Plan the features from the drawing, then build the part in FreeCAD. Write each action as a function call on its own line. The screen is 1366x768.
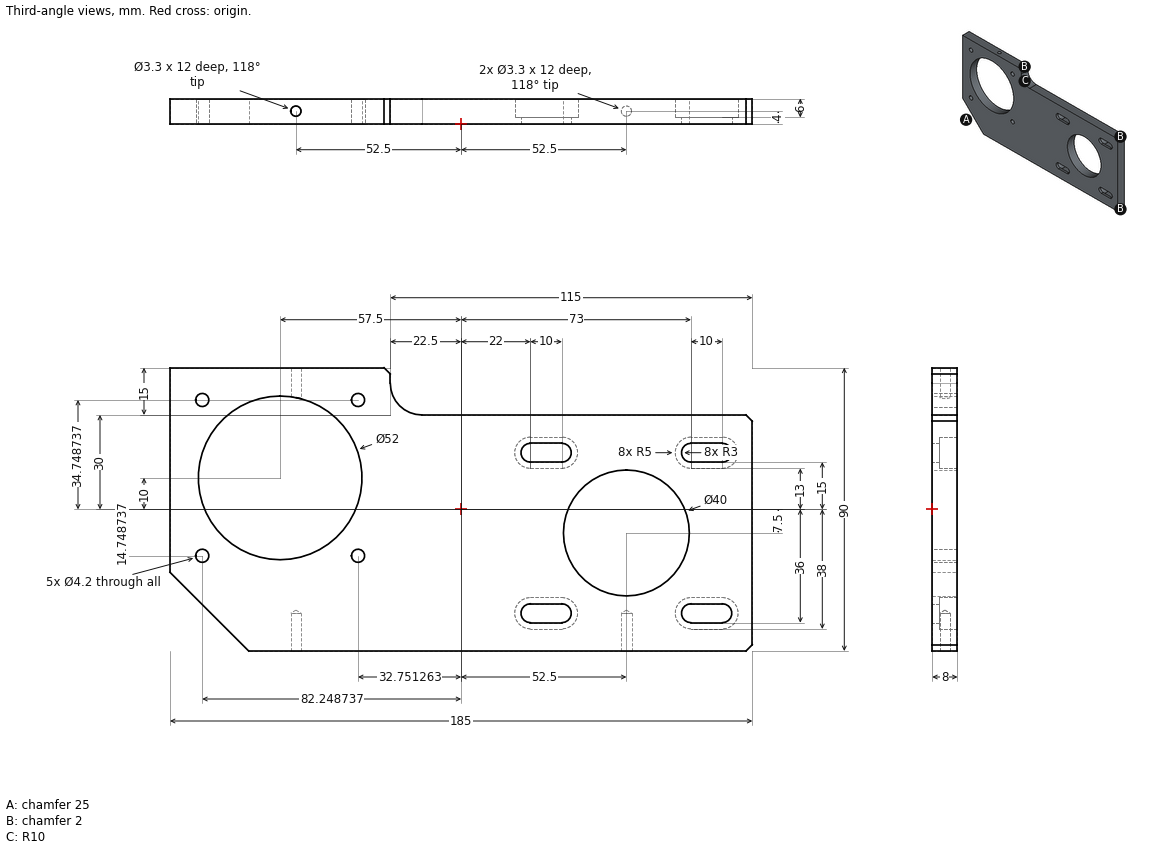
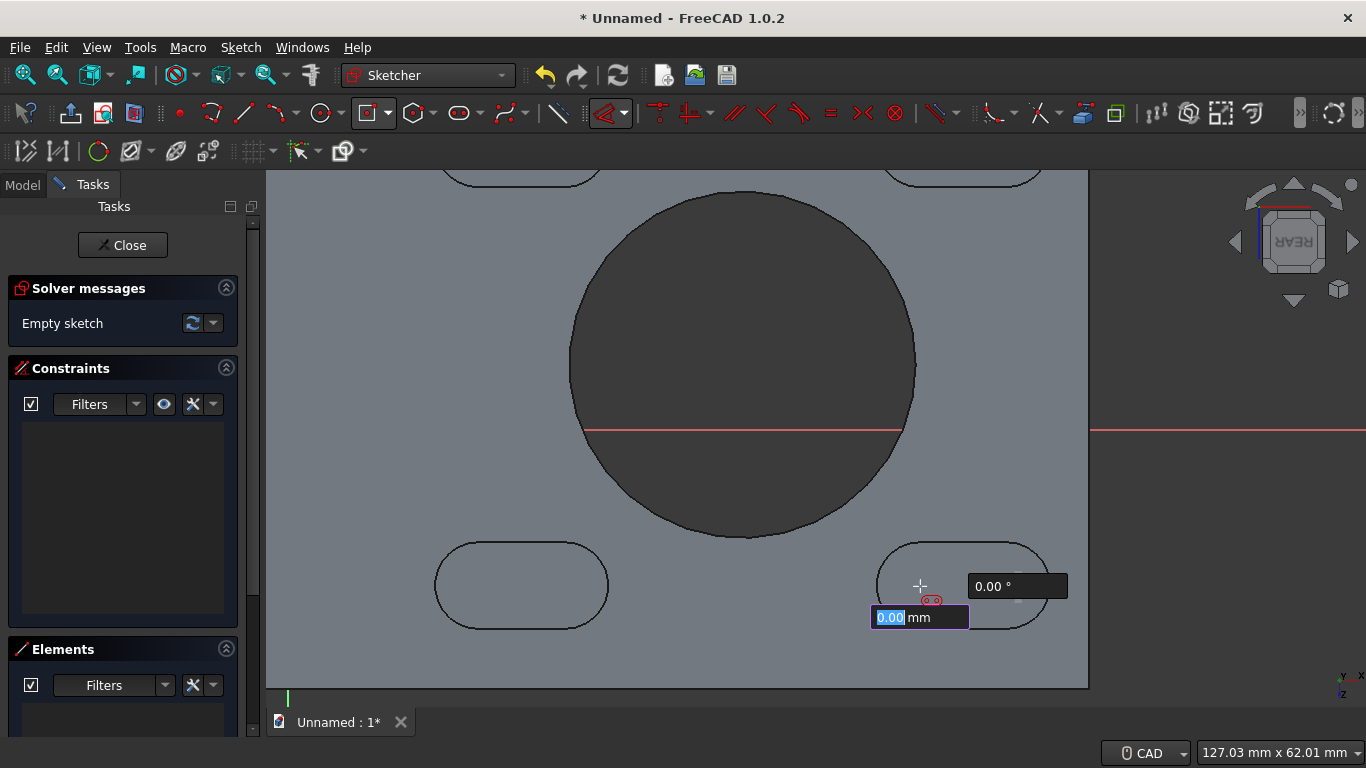
click(1007, 586)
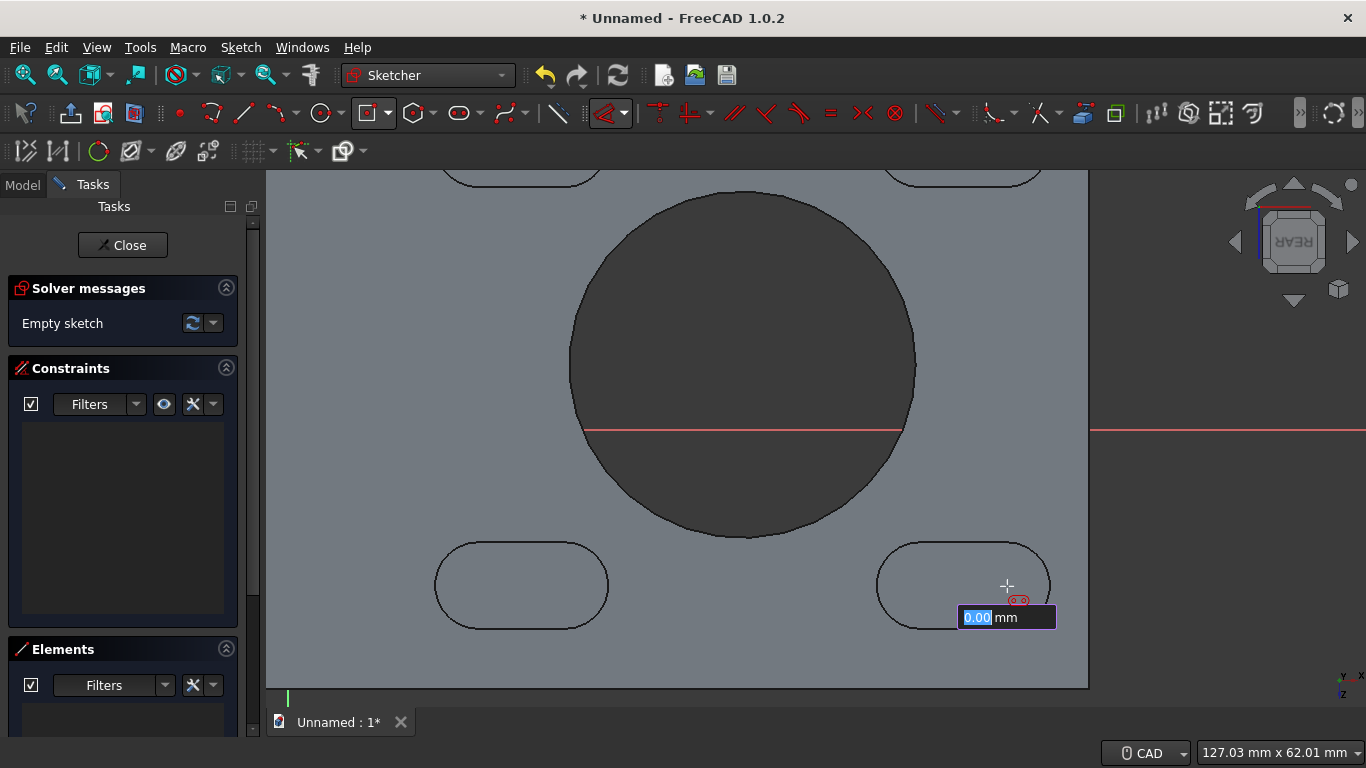
click(963, 560)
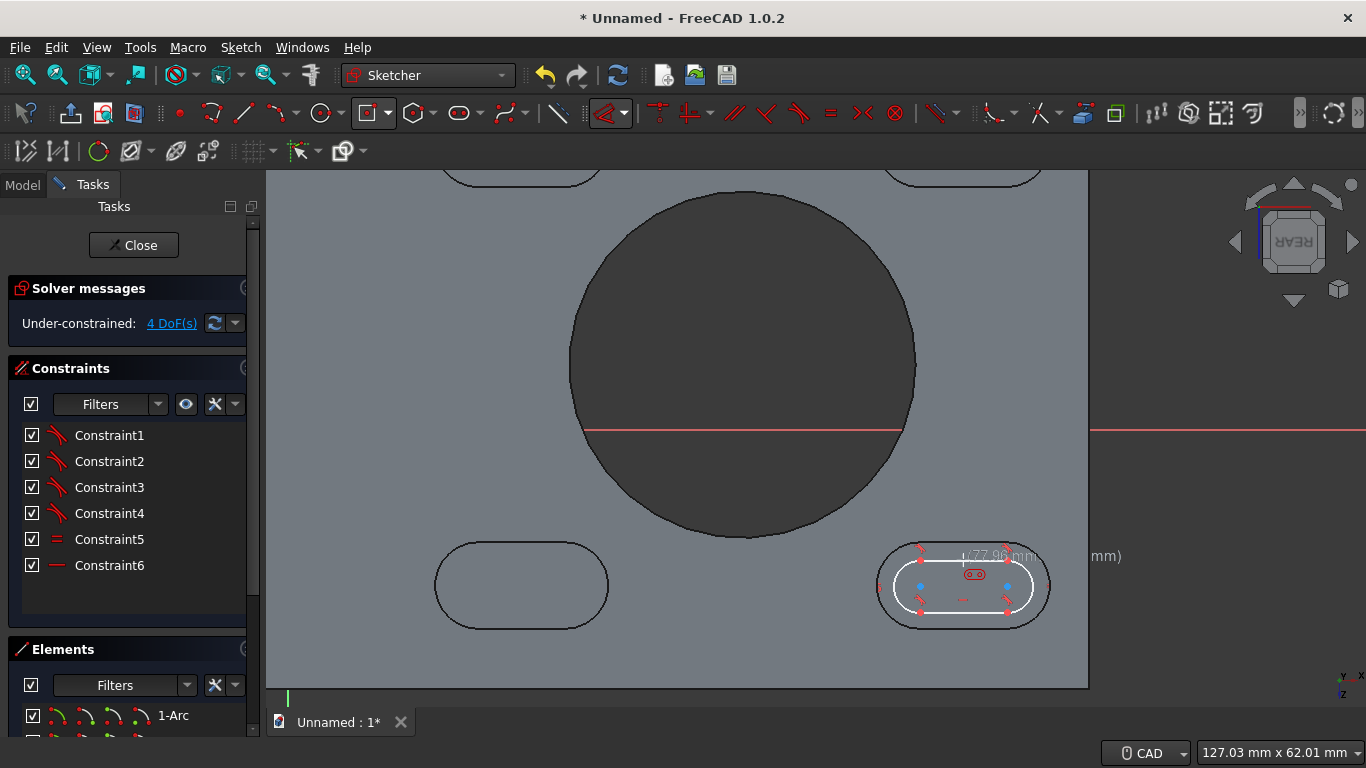
scroll(925, 588, down, 2)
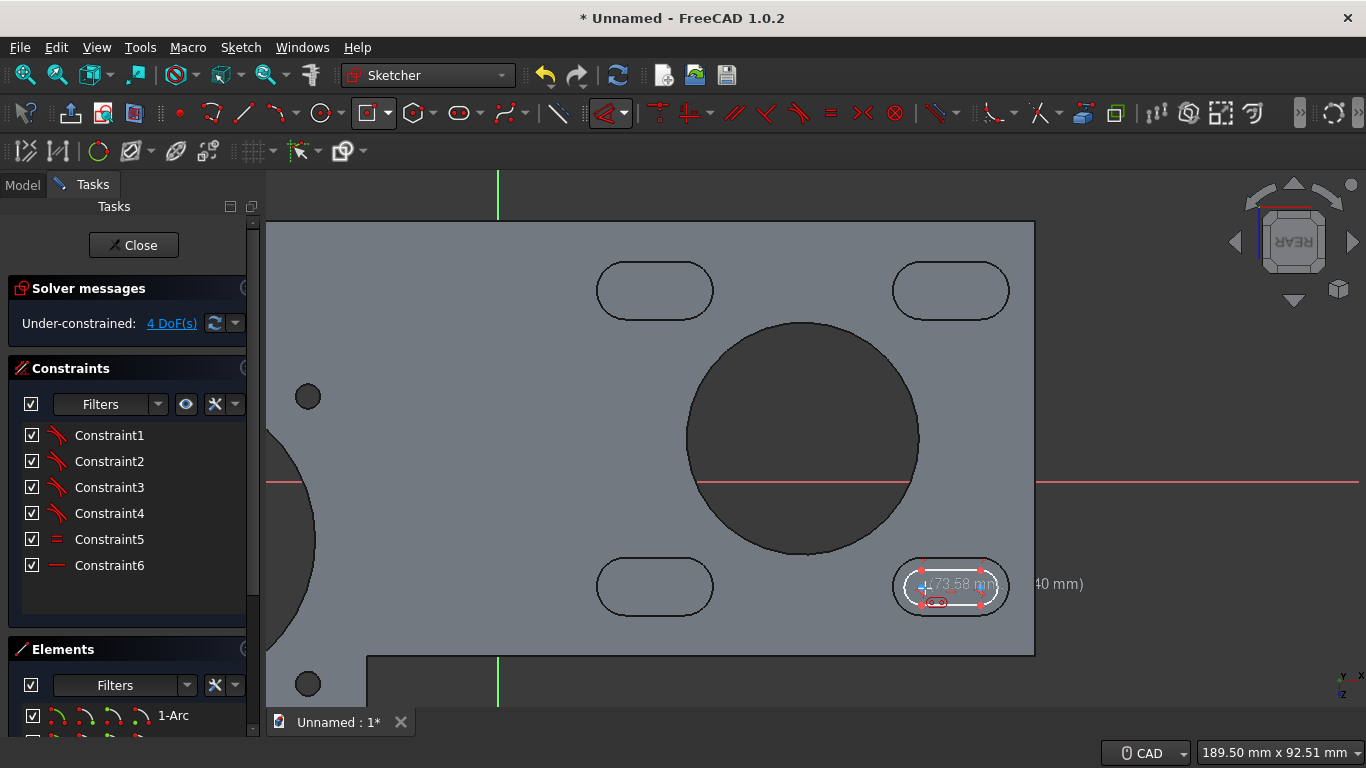
scroll(922, 291, up, 2)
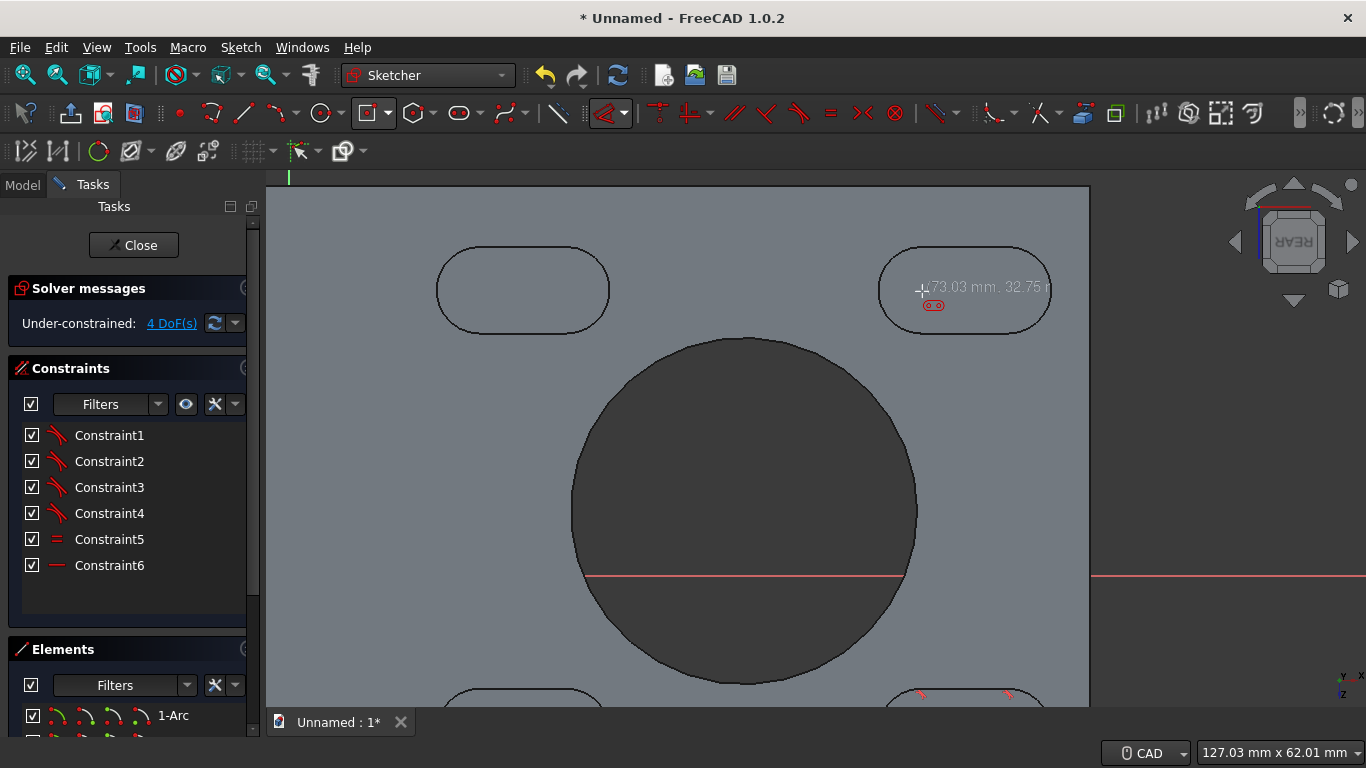
click(921, 290)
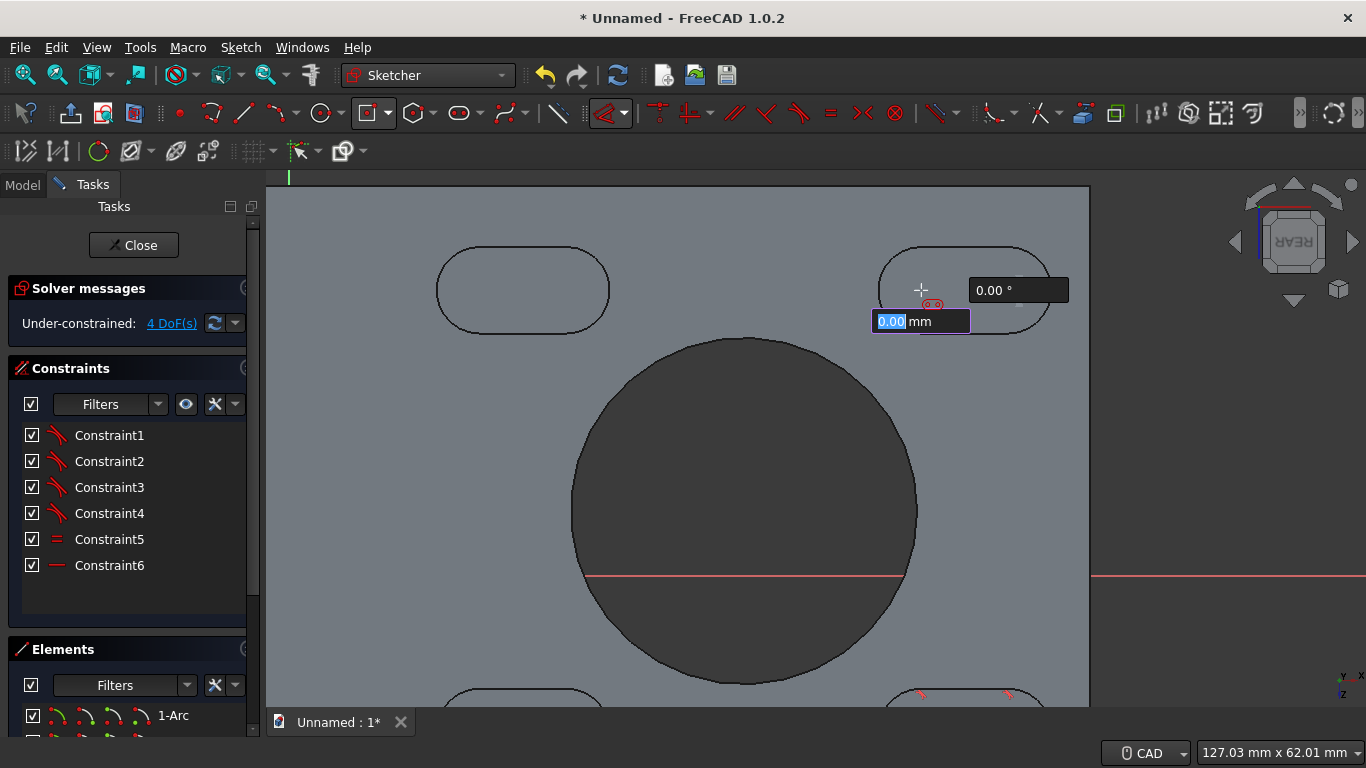
click(1008, 290)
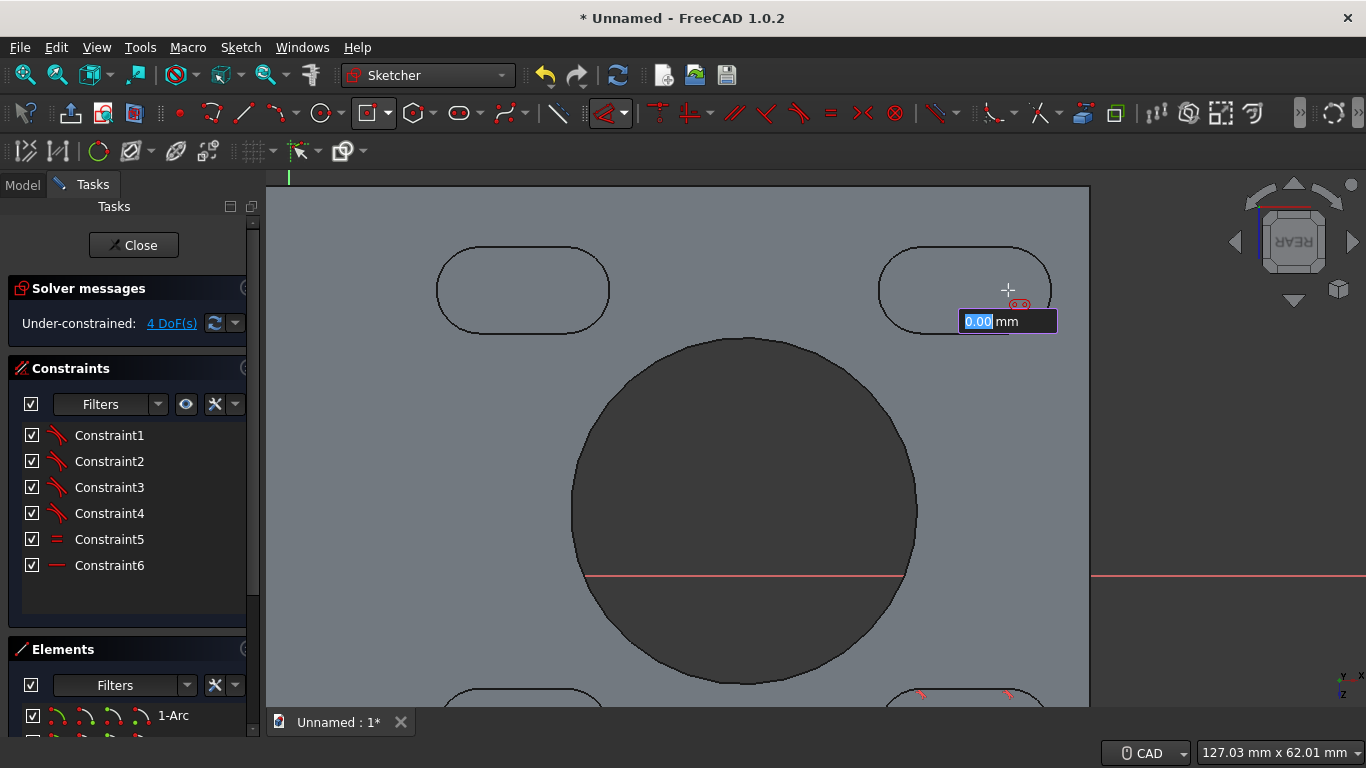
click(965, 316)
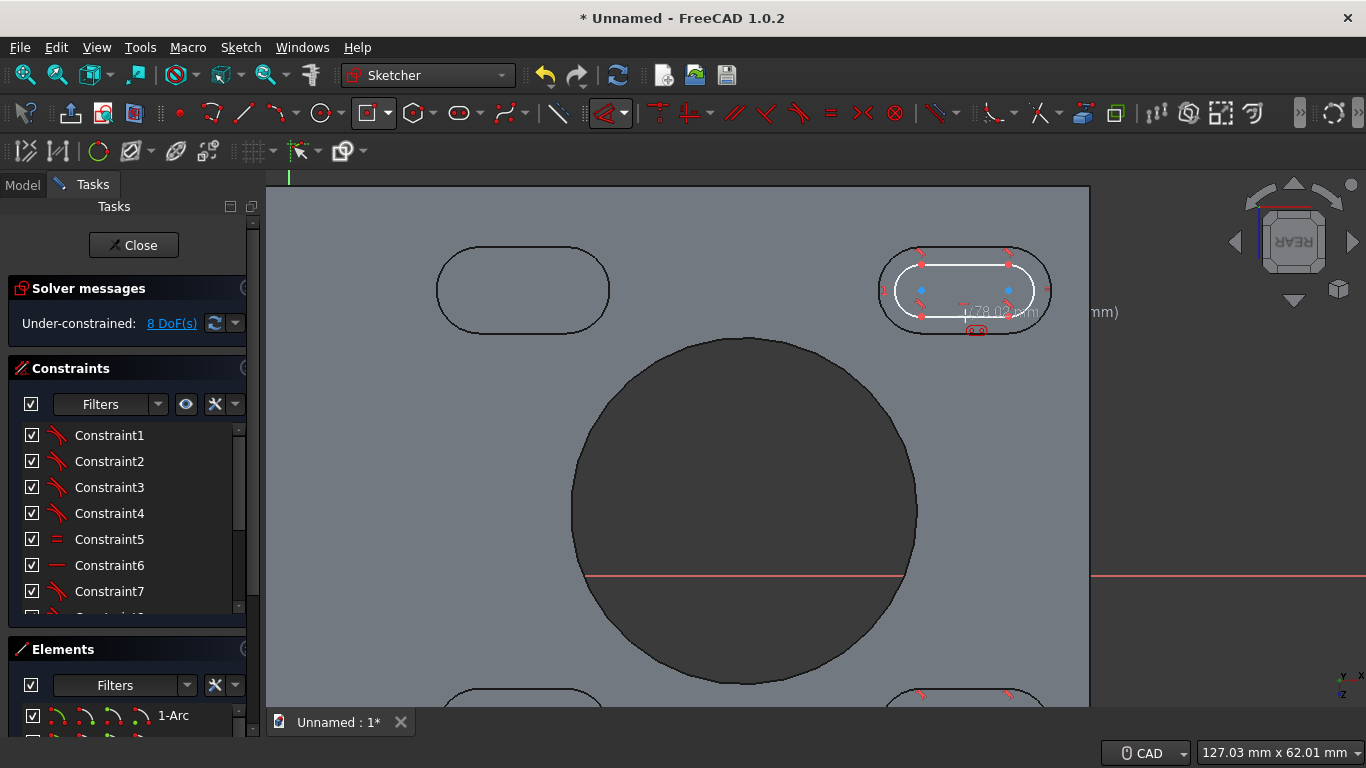
scroll(922, 291, down, 2)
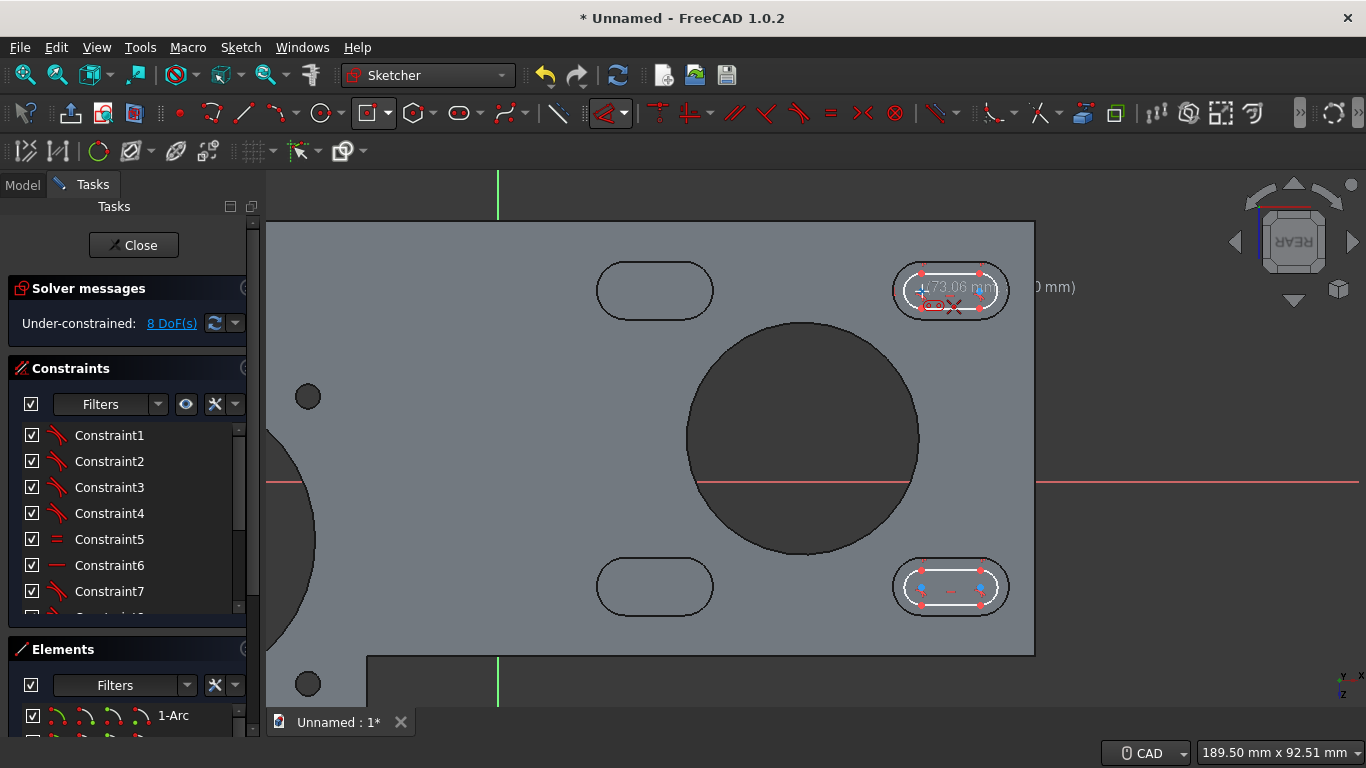
scroll(626, 587, up, 2)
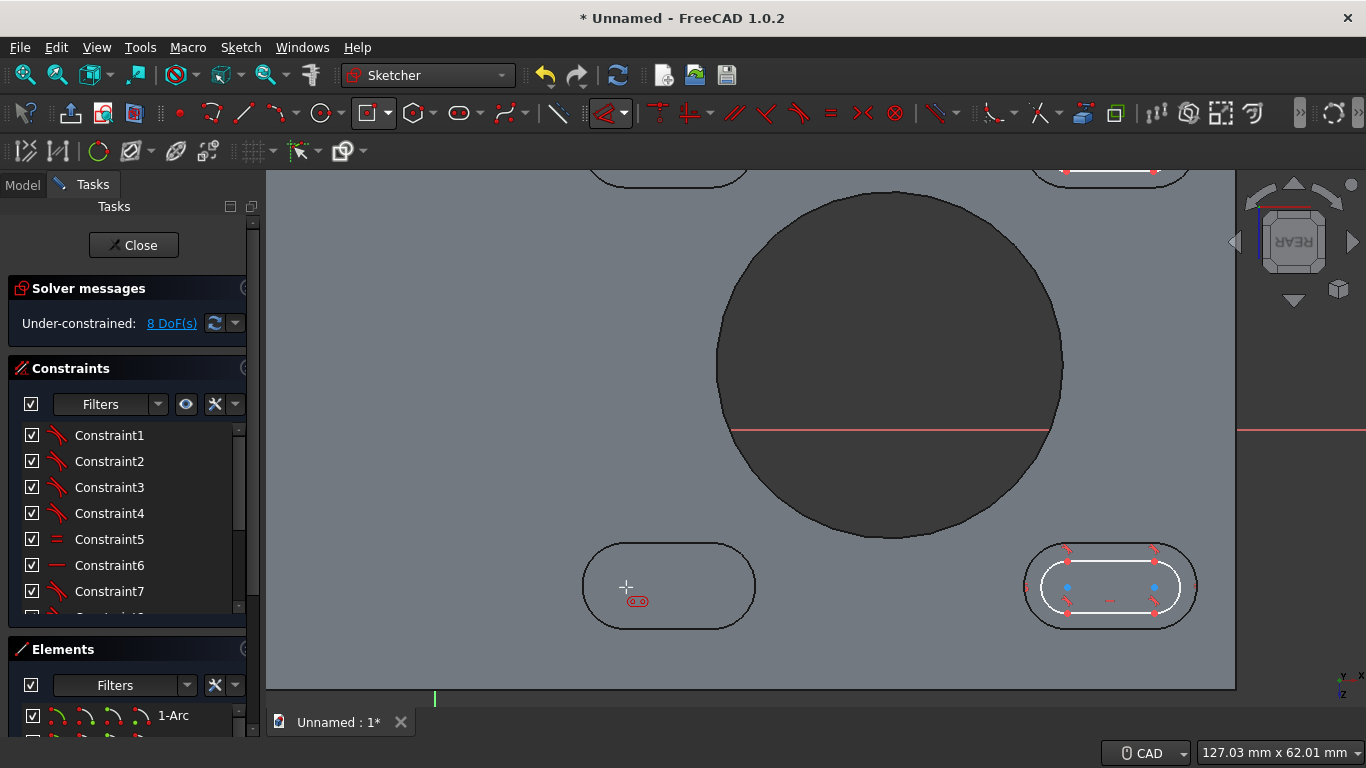
click(626, 586)